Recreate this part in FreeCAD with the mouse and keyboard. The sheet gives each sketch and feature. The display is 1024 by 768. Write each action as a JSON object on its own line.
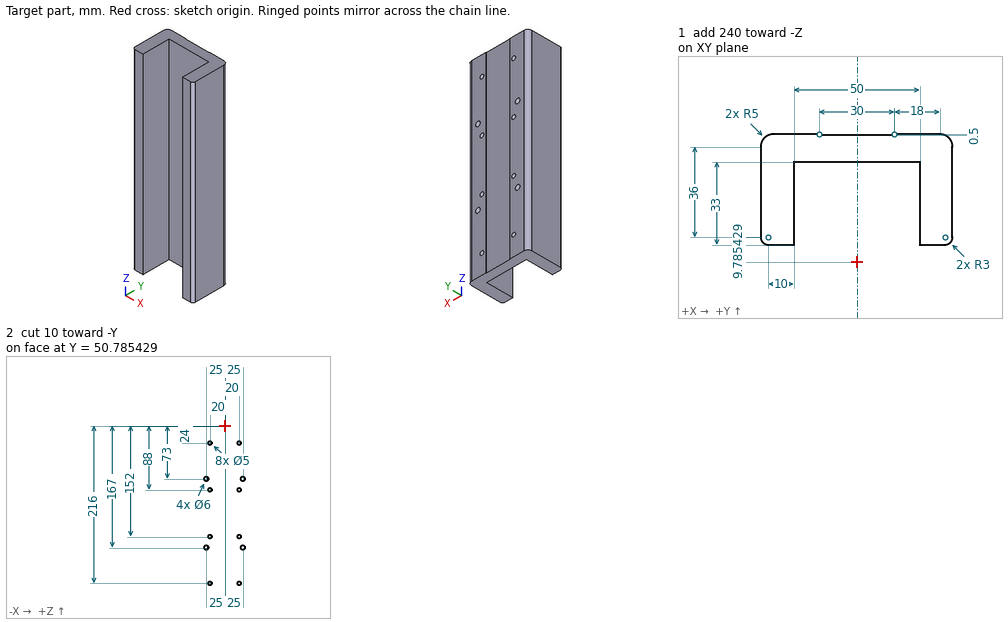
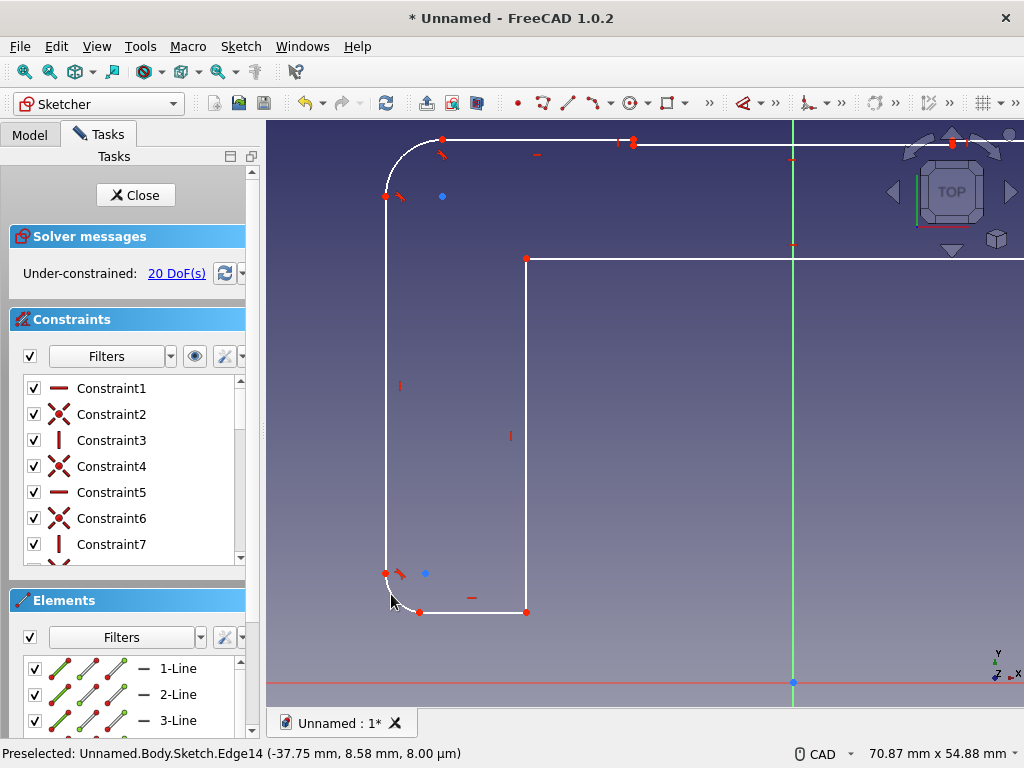
{"action": "left_click", "coordinate": [451, 613]}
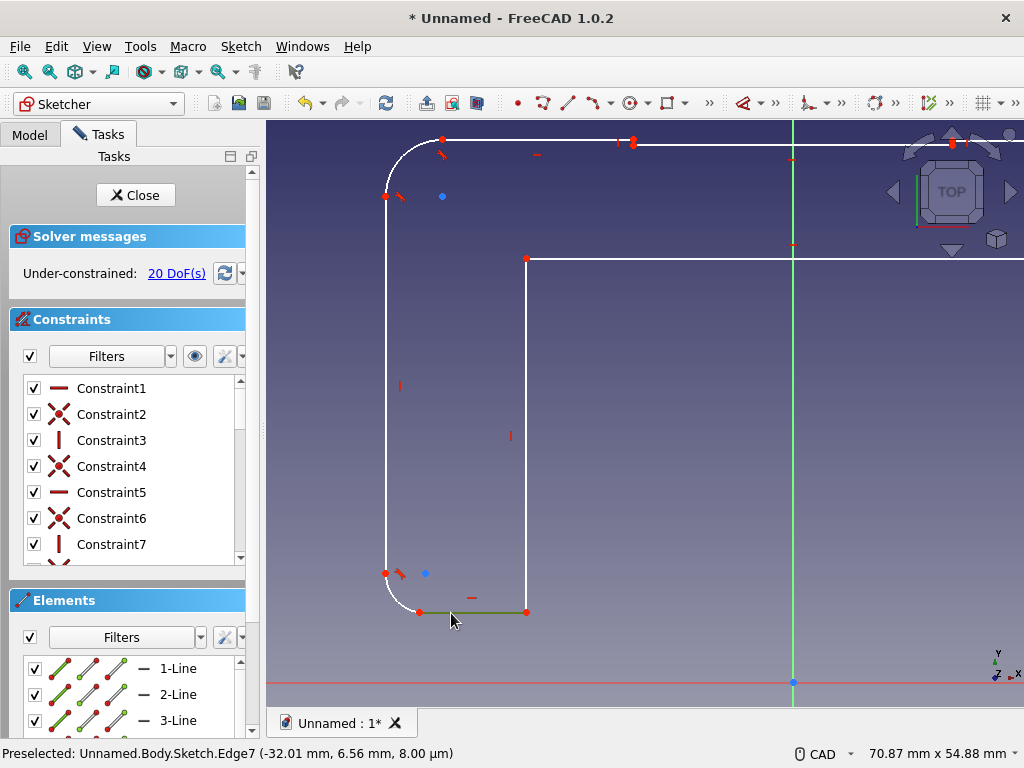
{"action": "left_click", "coordinate": [389, 590]}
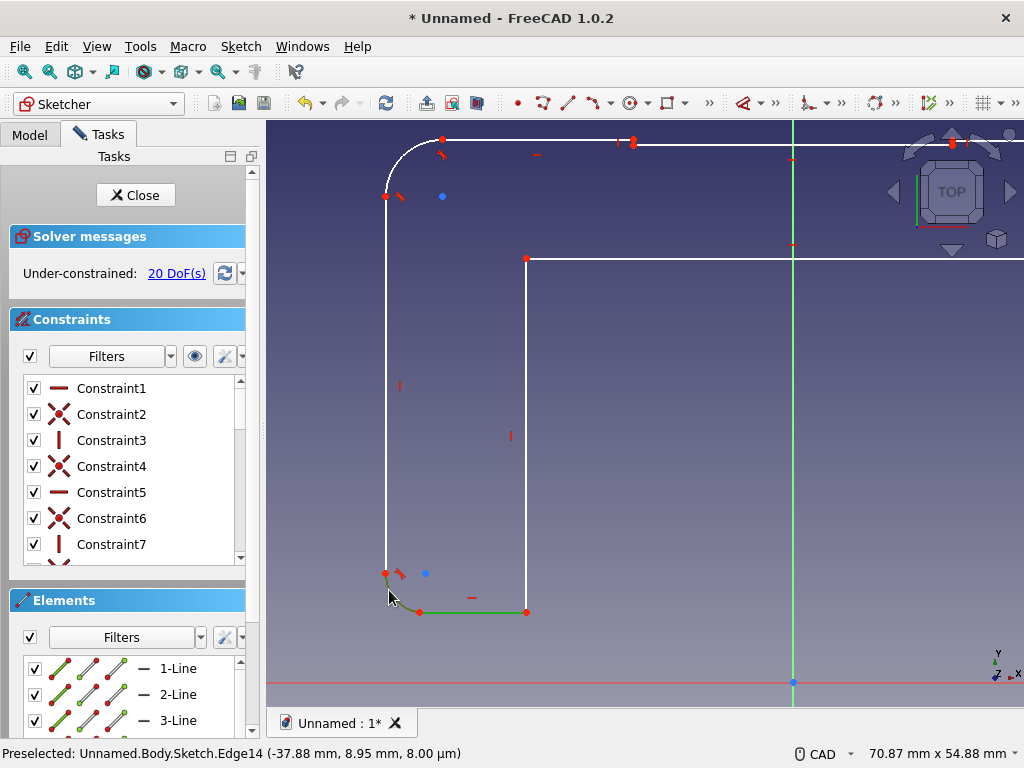
{"action": "key", "text": "t"}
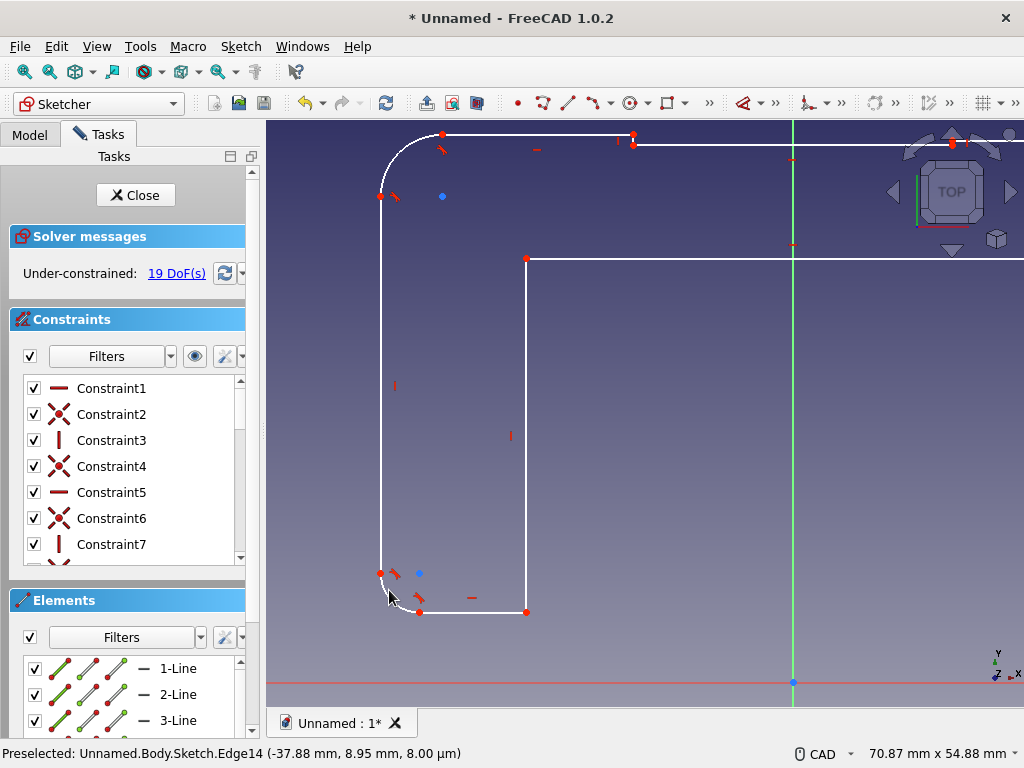
{"action": "scroll", "coordinate": [400, 415], "scroll_direction": "down", "scroll_amount": 4}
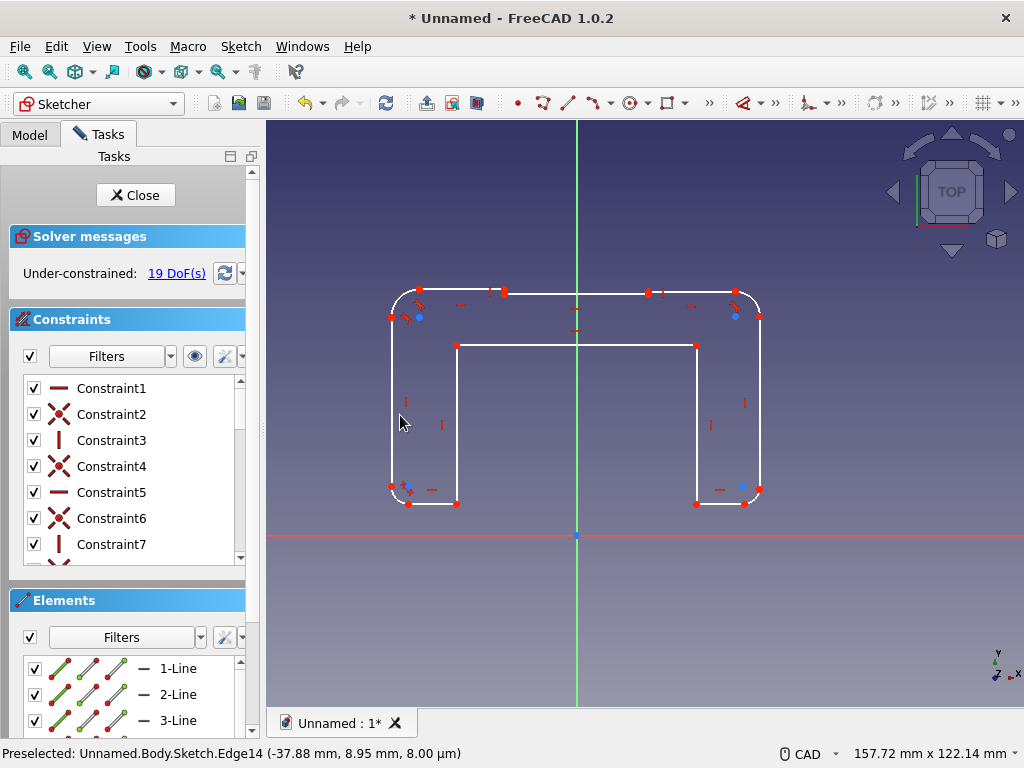
{"action": "left_click", "coordinate": [711, 504]}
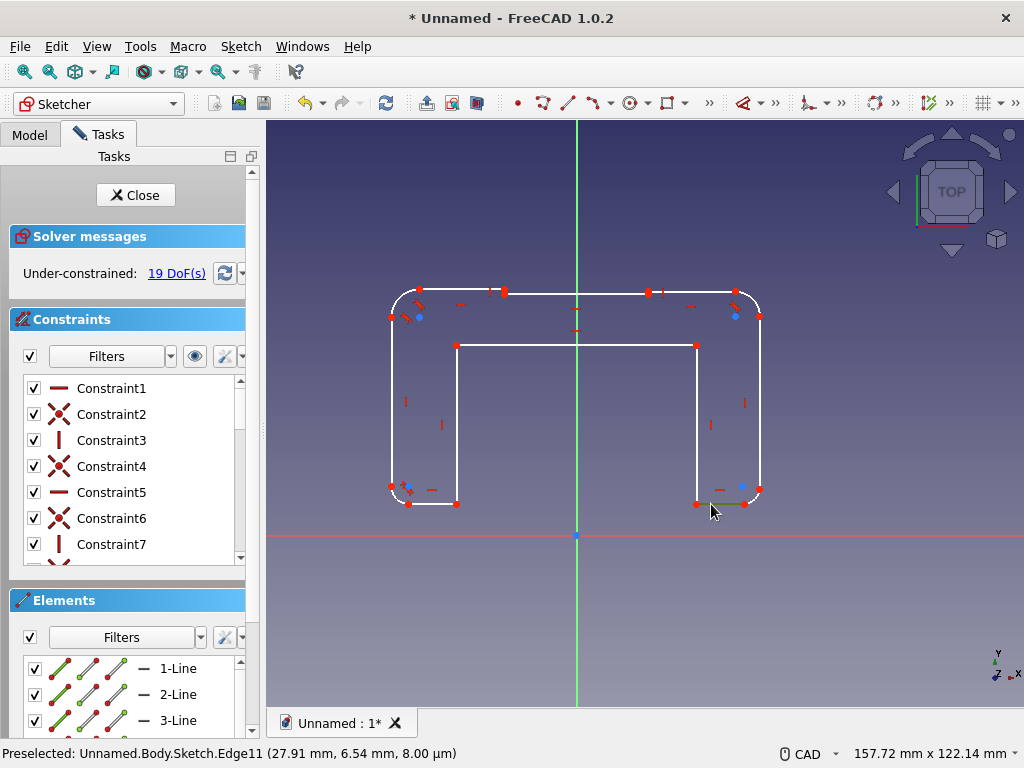
{"action": "scroll", "coordinate": [755, 499], "scroll_direction": "up", "scroll_amount": 2}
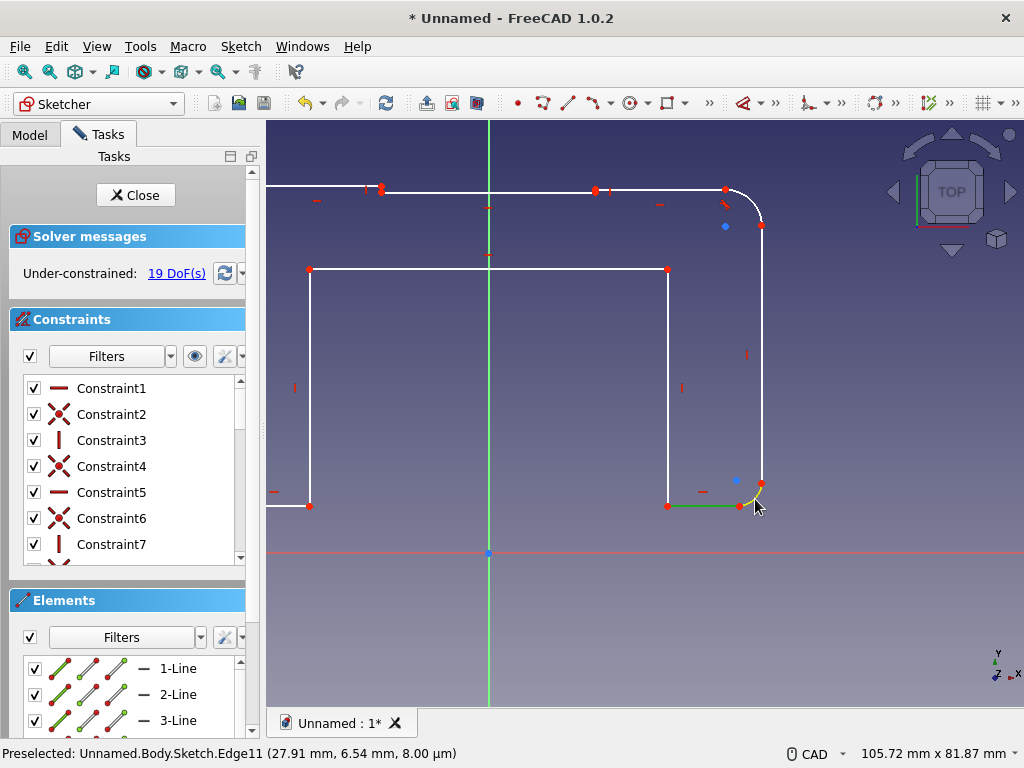
{"action": "left_click", "coordinate": [754, 499]}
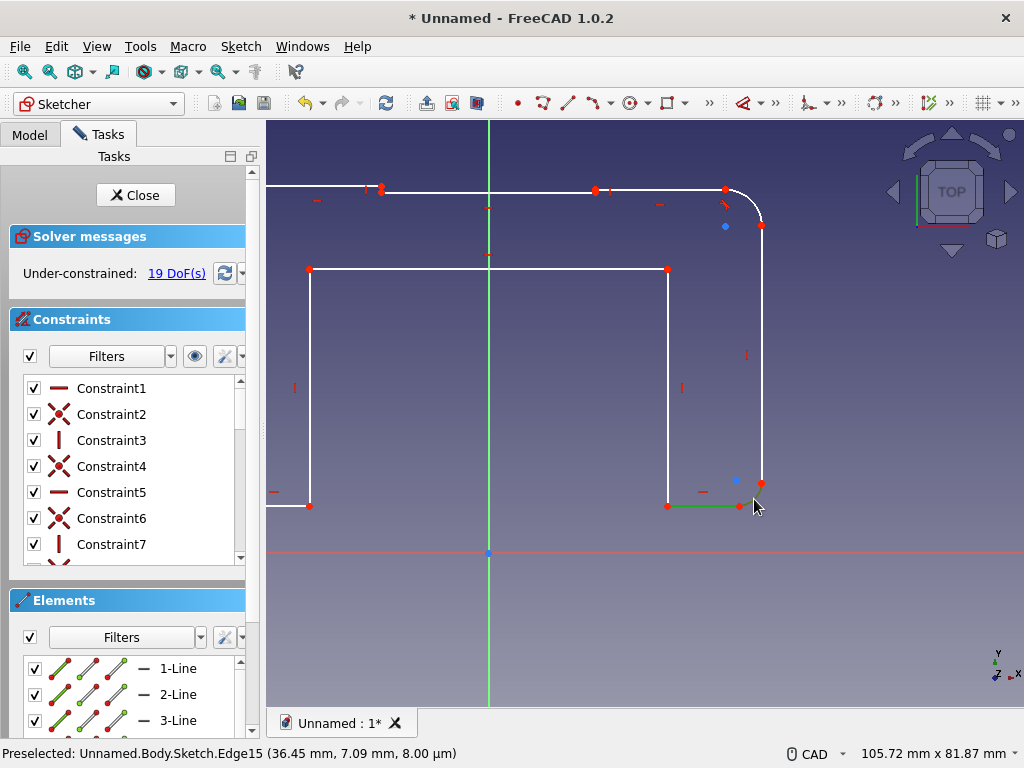
{"action": "key", "text": "t"}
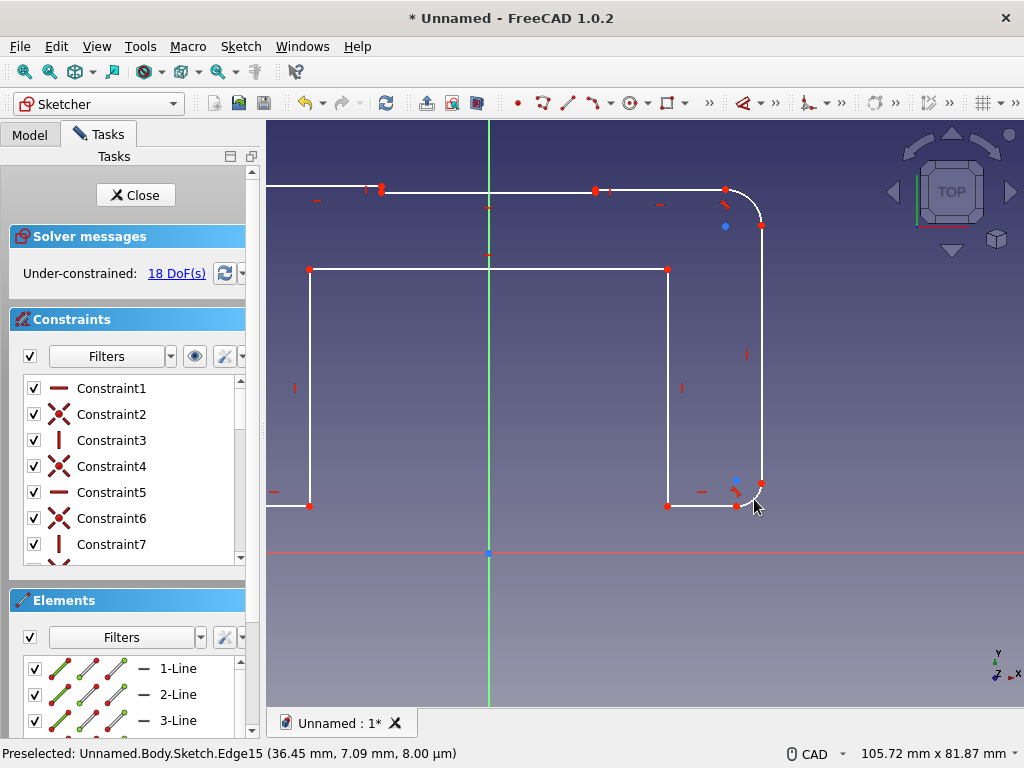
{"action": "left_click", "coordinate": [762, 407]}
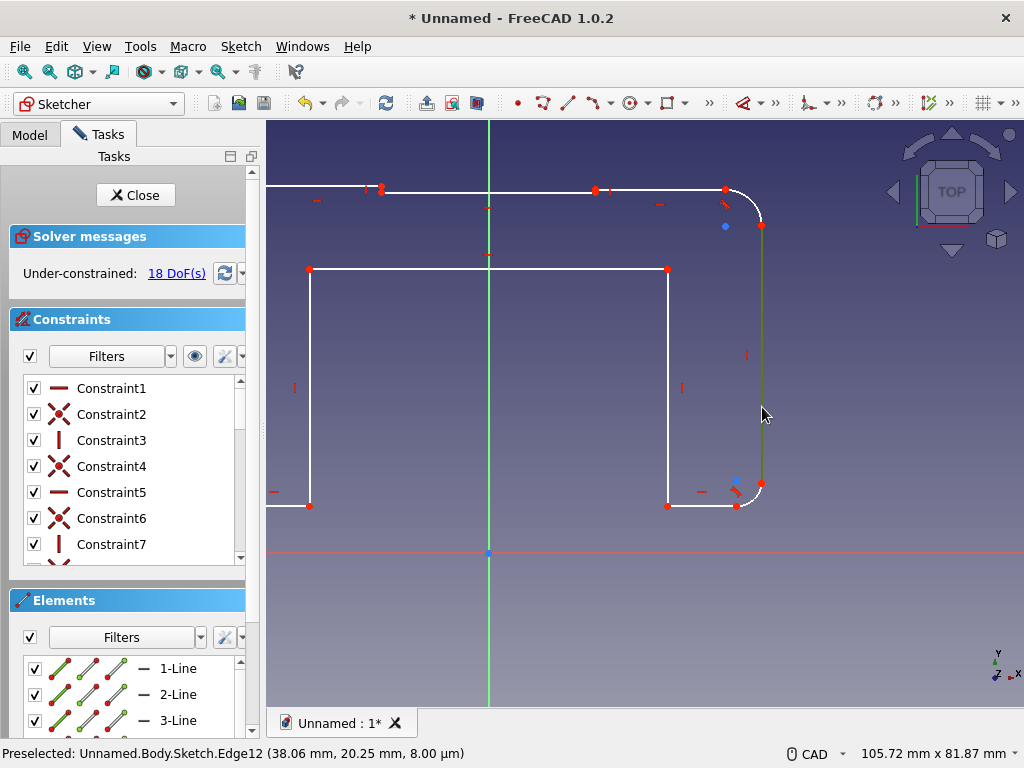
{"action": "scroll", "coordinate": [747, 504], "scroll_direction": "up", "scroll_amount": 2}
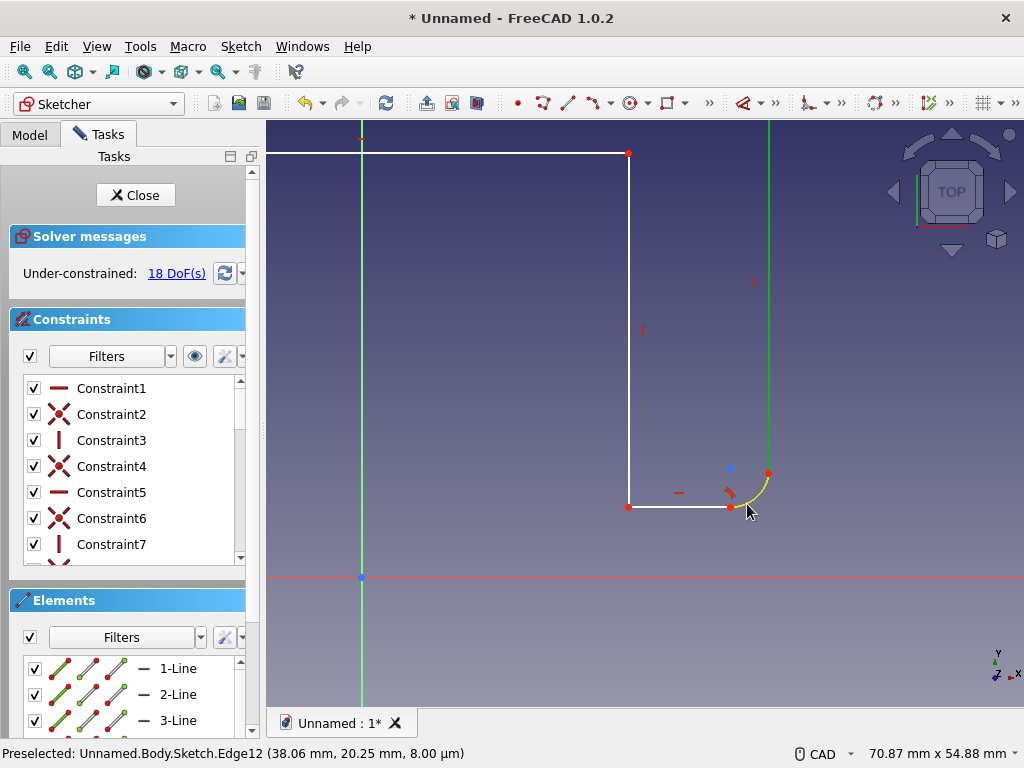
{"action": "left_click", "coordinate": [747, 504]}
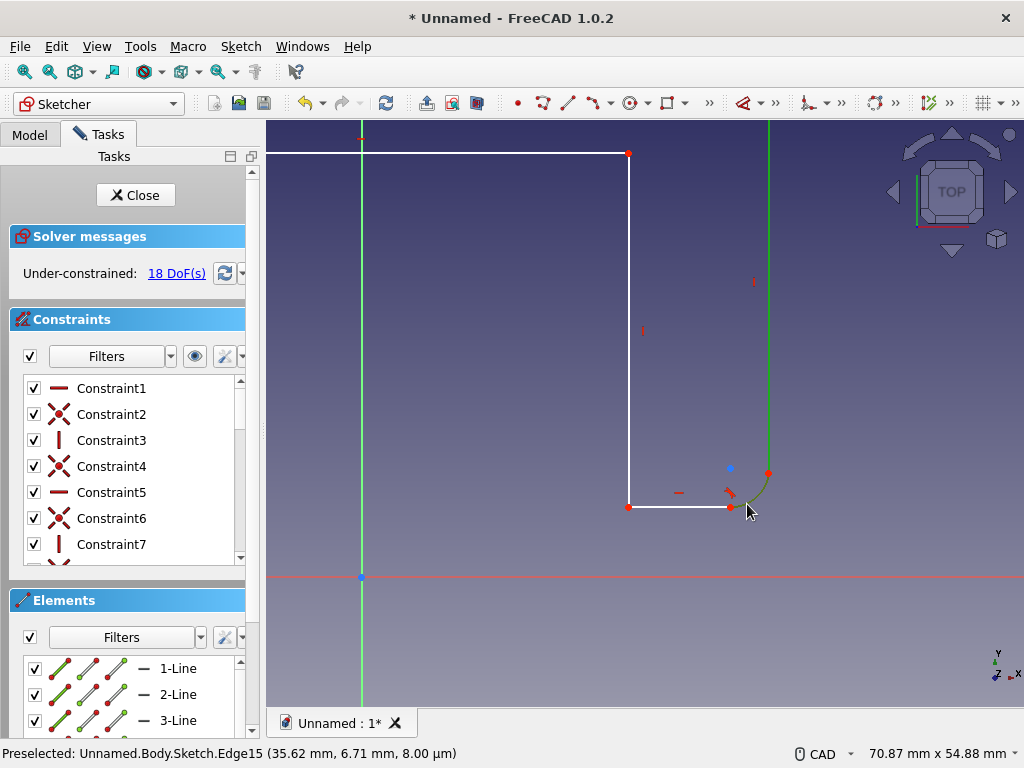
{"action": "key", "text": "t"}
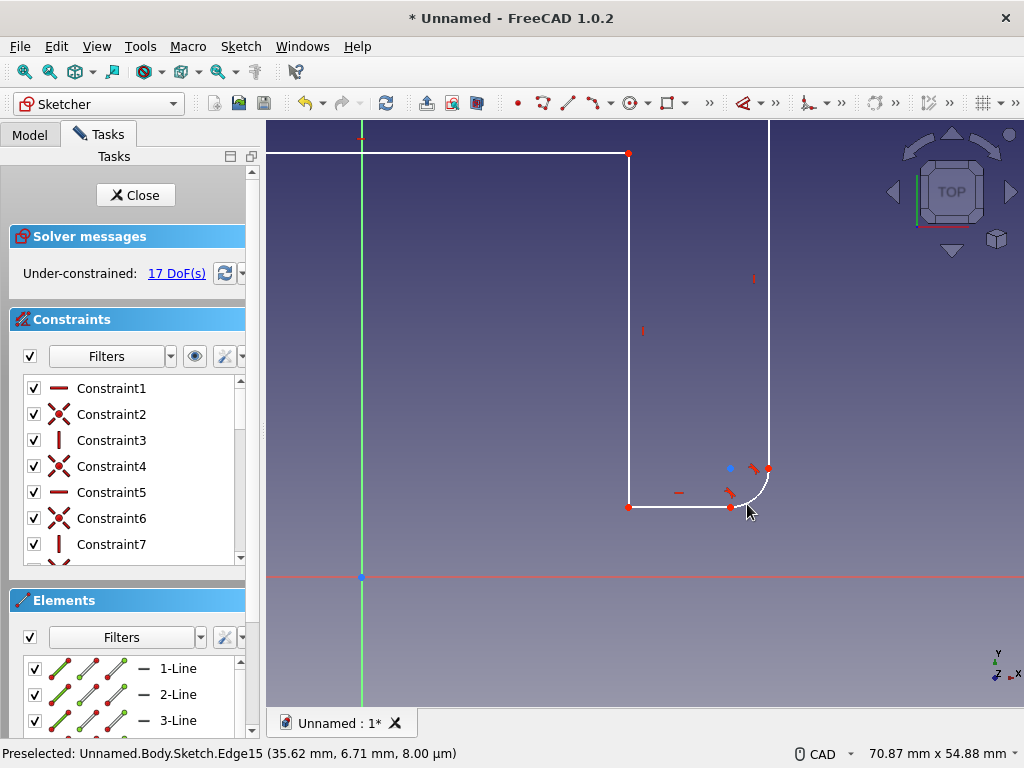
{"action": "left_click", "coordinate": [769, 355]}